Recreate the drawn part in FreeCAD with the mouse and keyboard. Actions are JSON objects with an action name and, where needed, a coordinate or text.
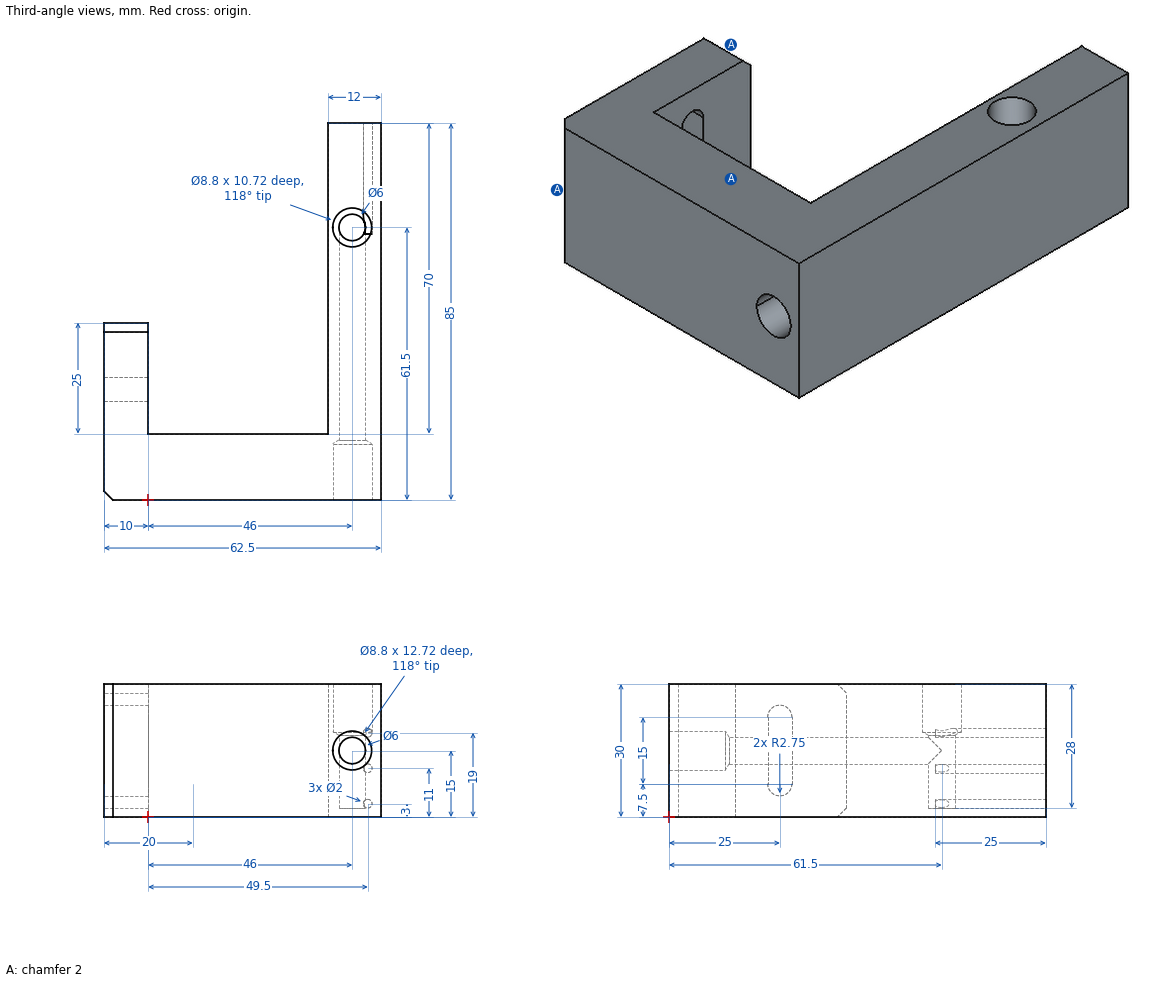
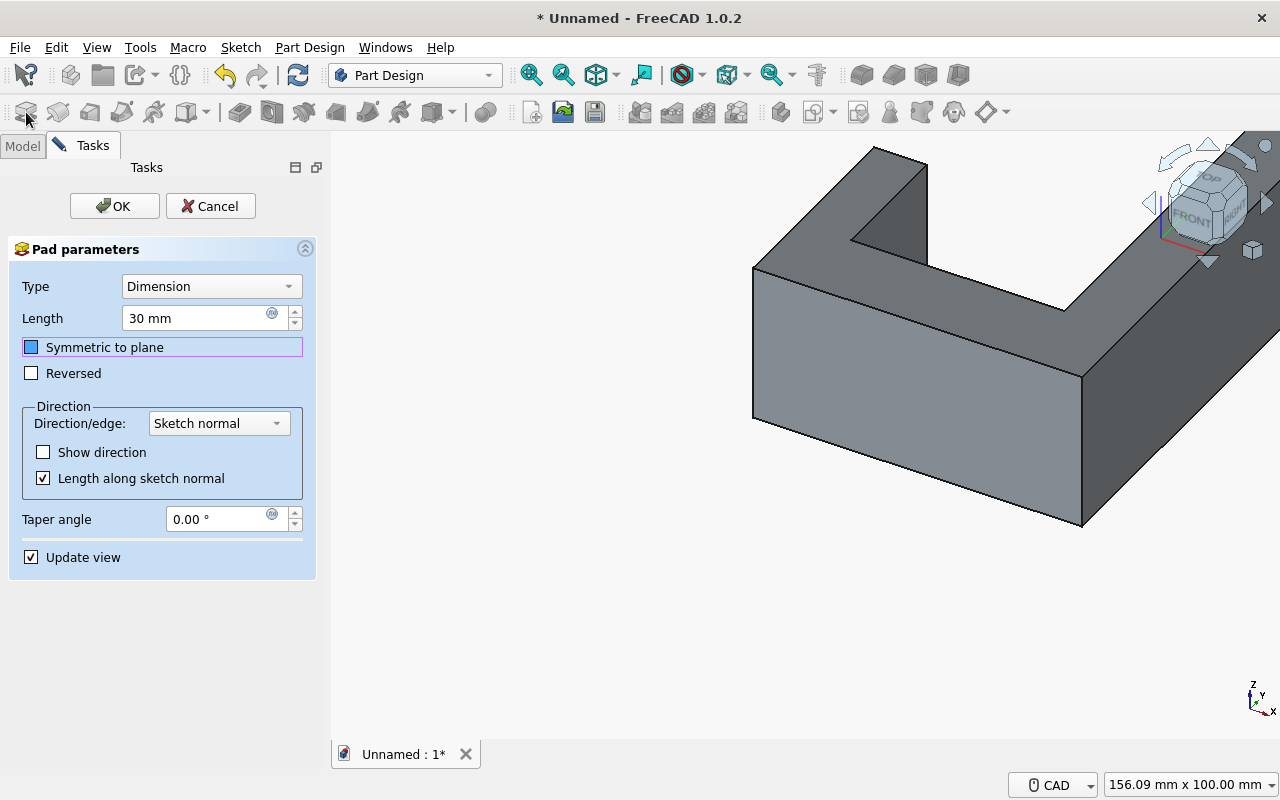
{"action": "left_click", "coordinate": [115, 206]}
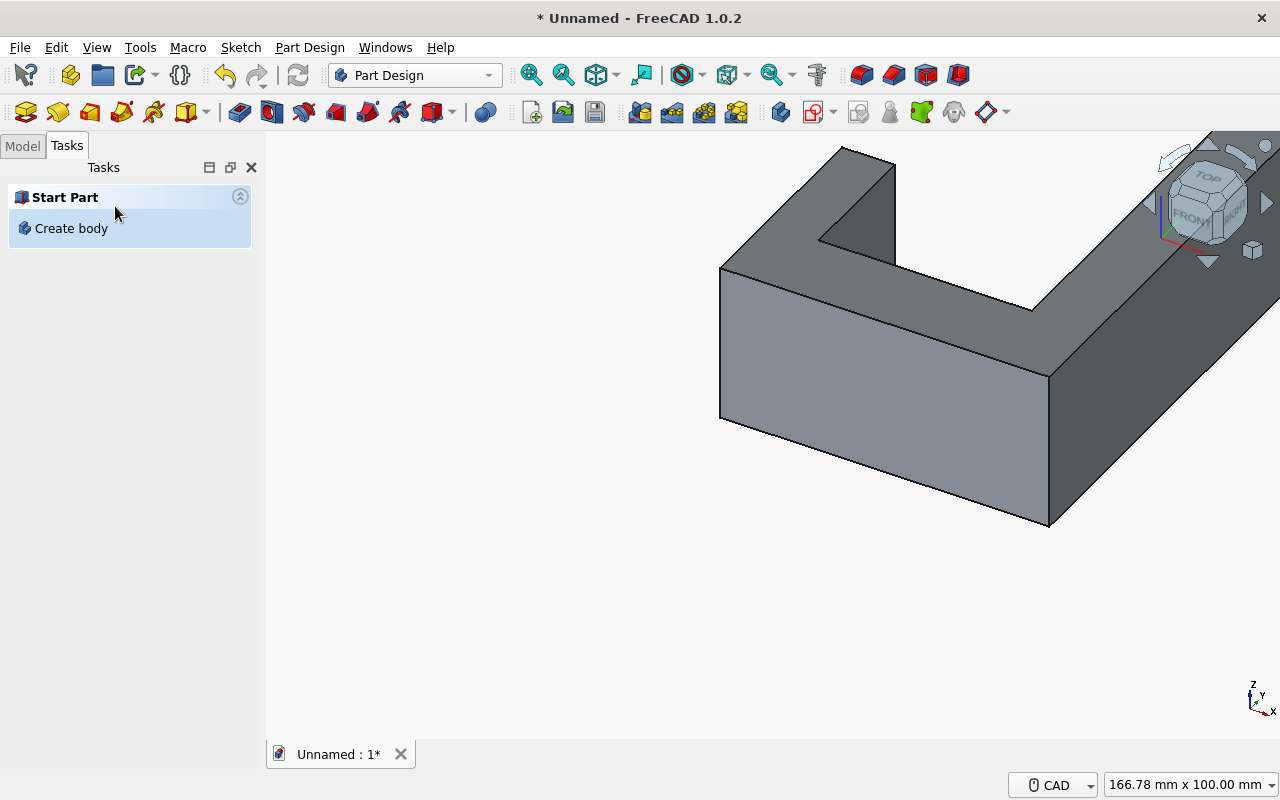
{"action": "key", "text": "v f"}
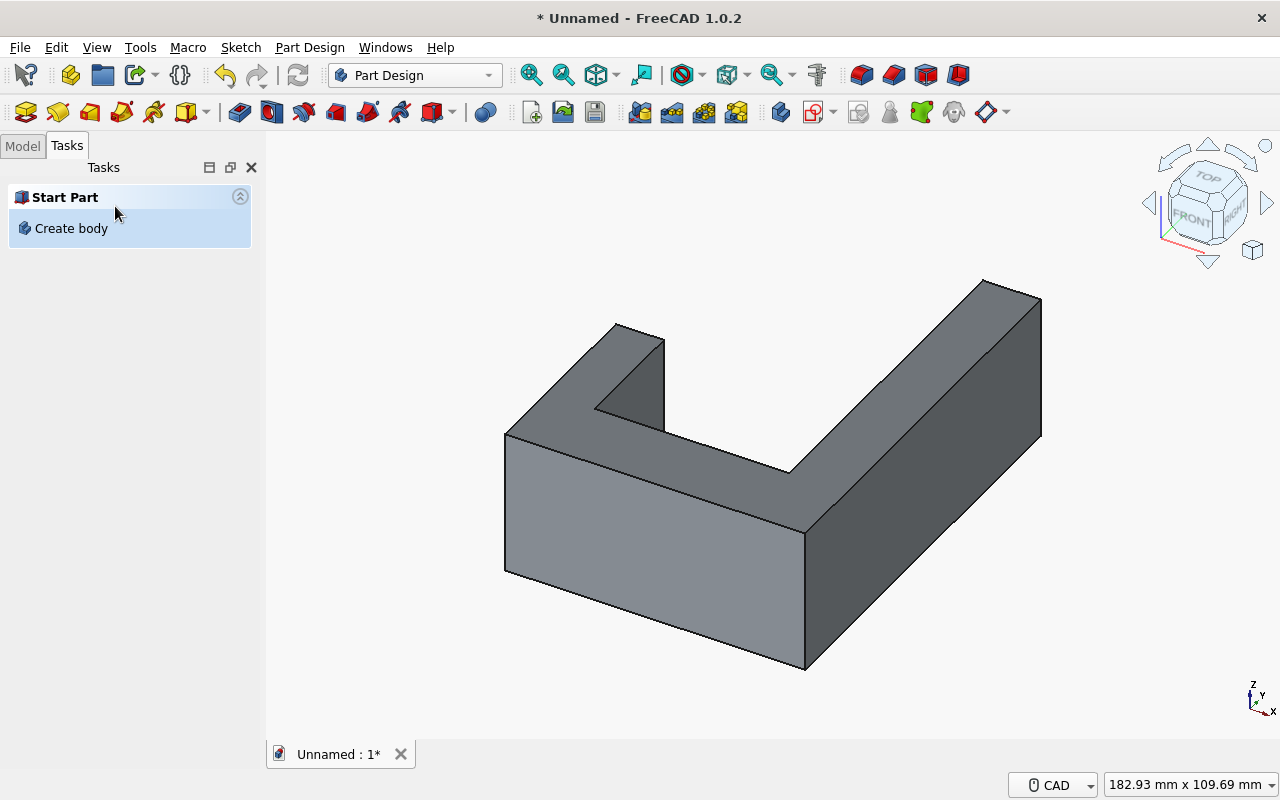
{"action": "key", "text": "4"}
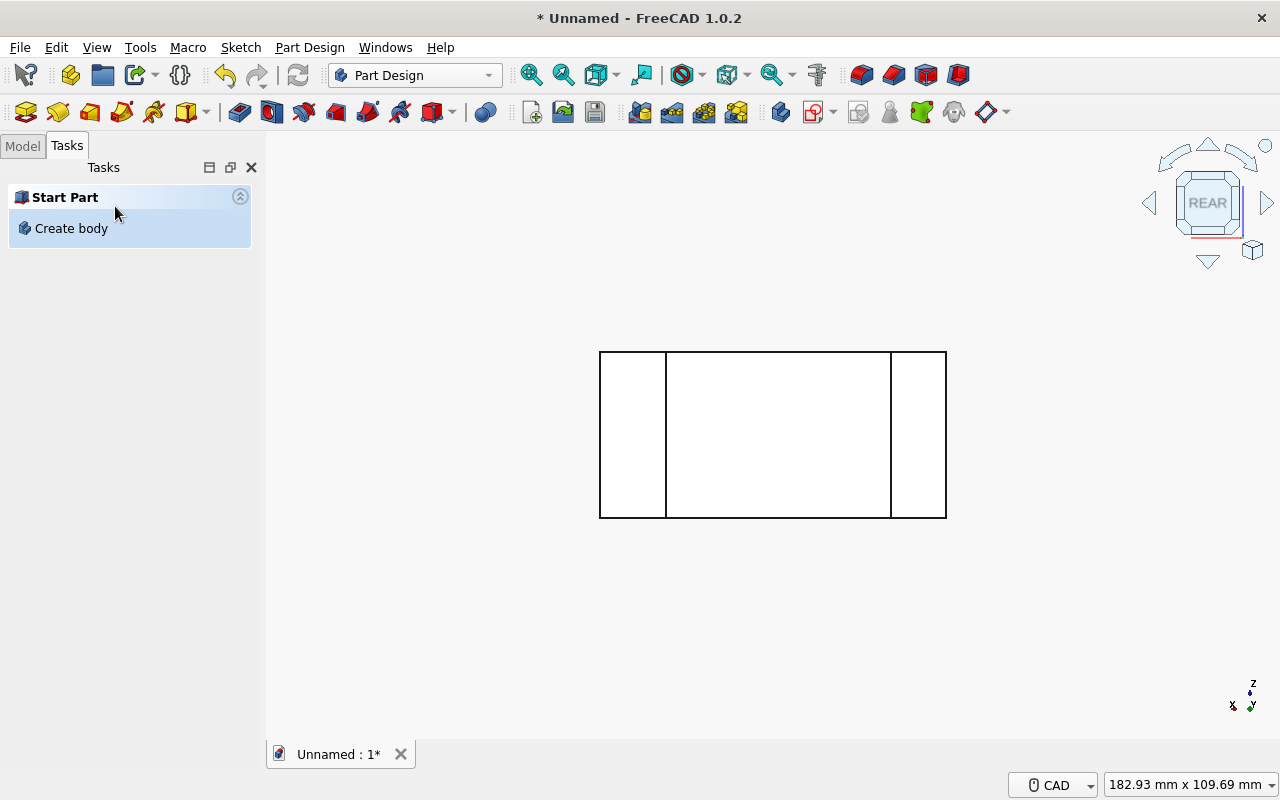
{"action": "key", "text": "v f"}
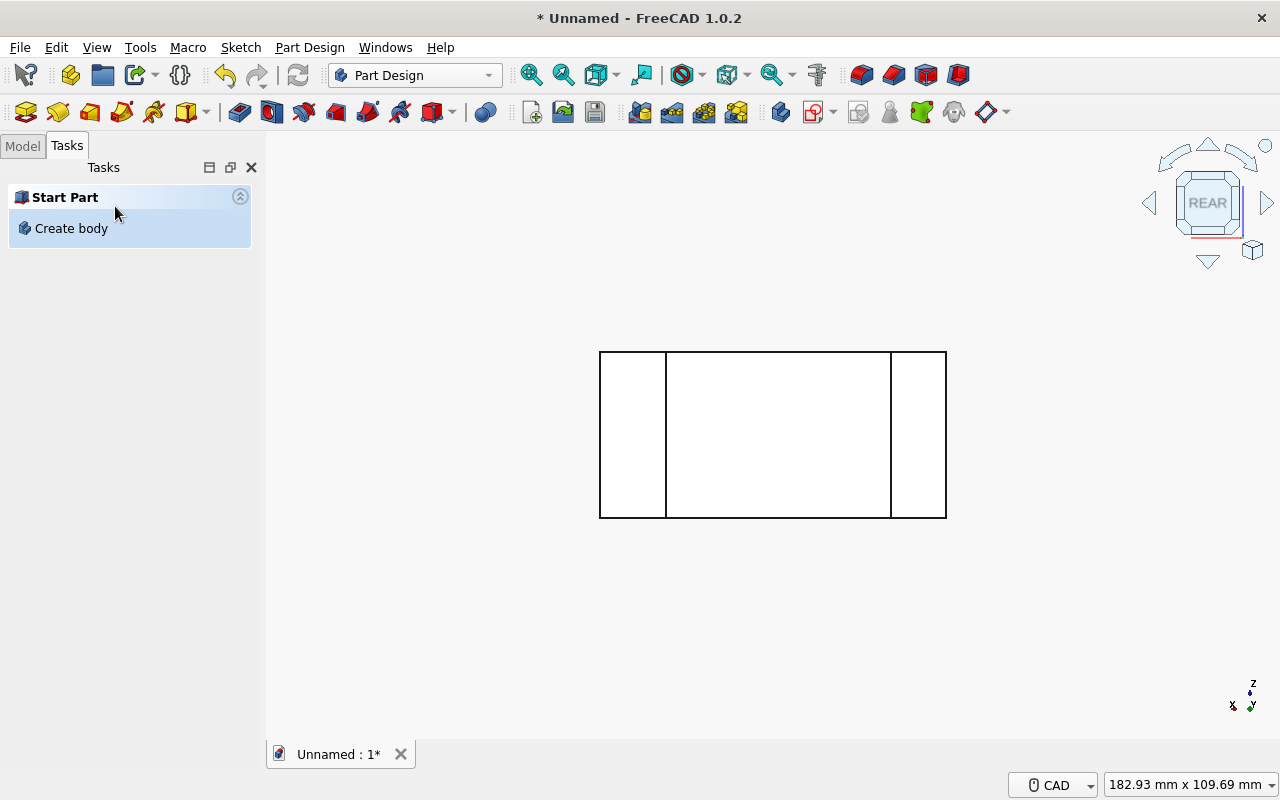
{"action": "left_click", "coordinate": [633, 386]}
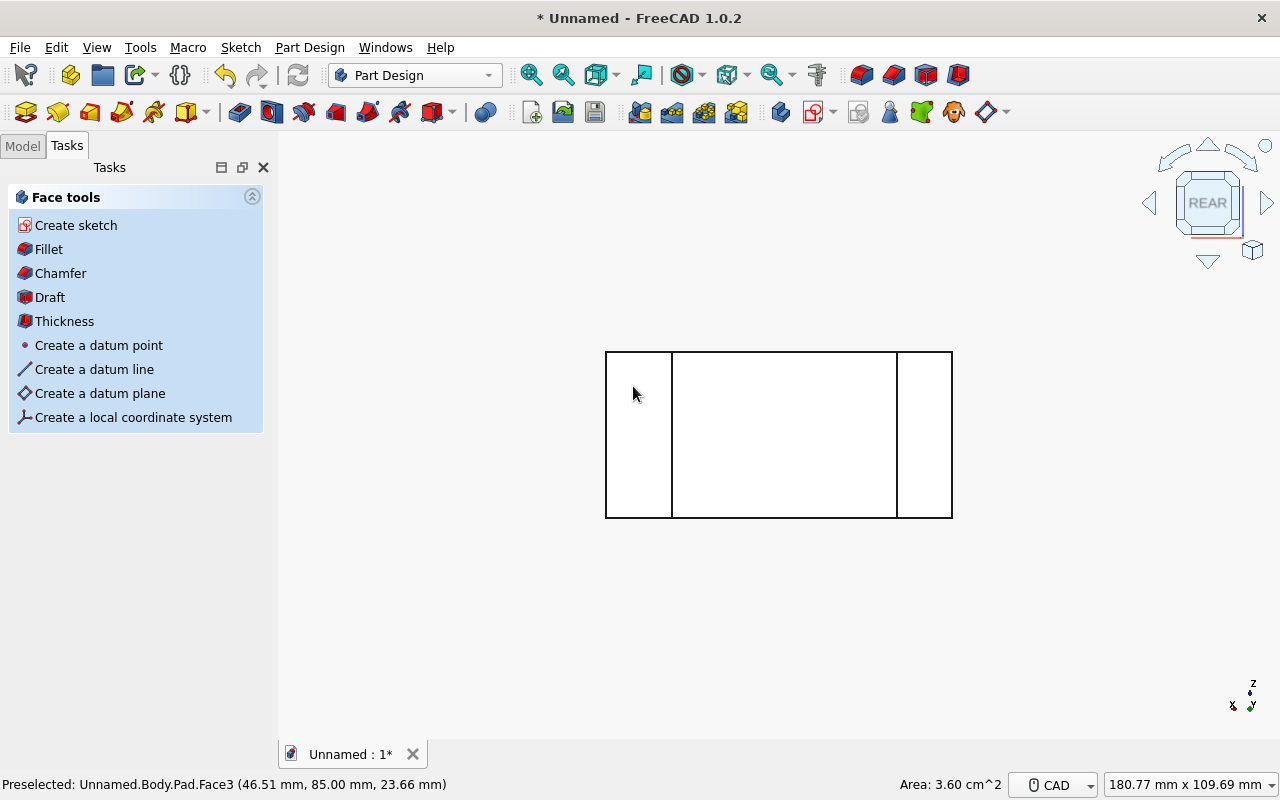
{"action": "left_click", "coordinate": [814, 112]}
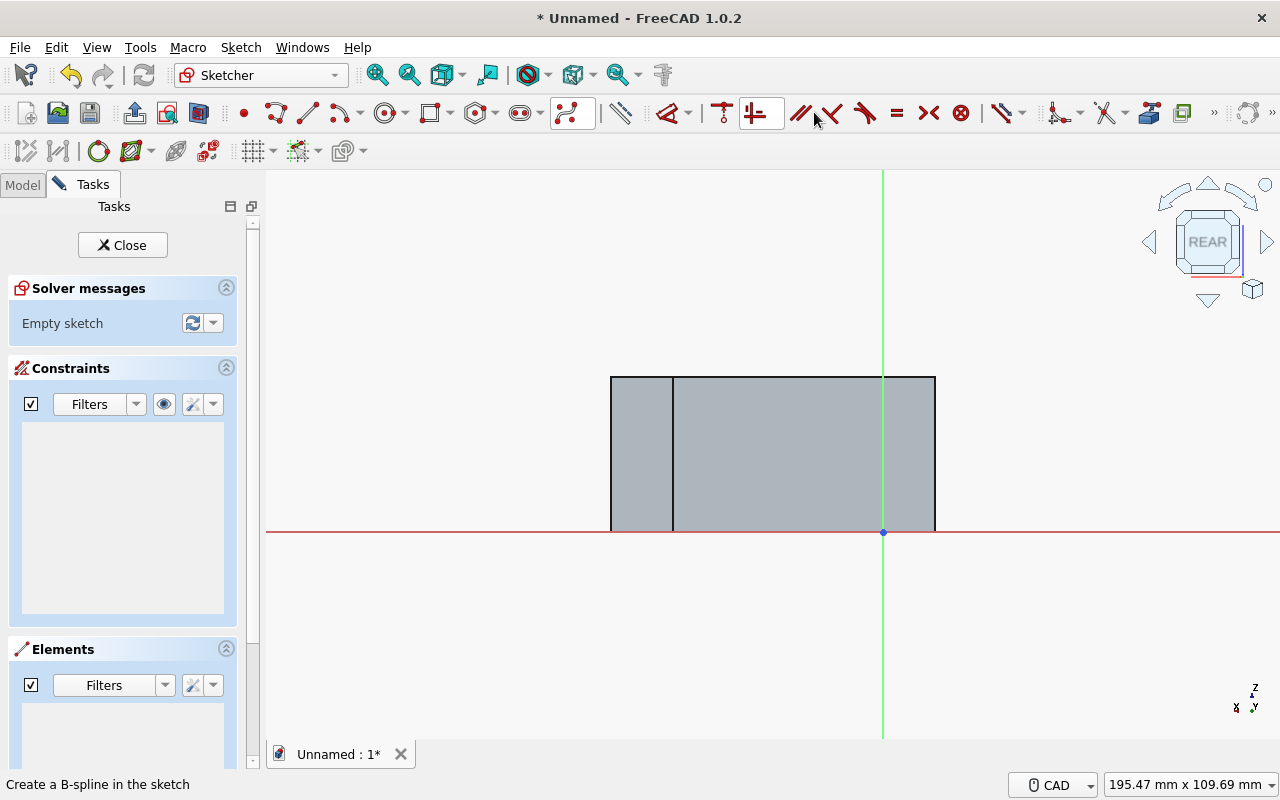
{"action": "scroll", "coordinate": [601, 482], "scroll_direction": "up", "scroll_amount": 7}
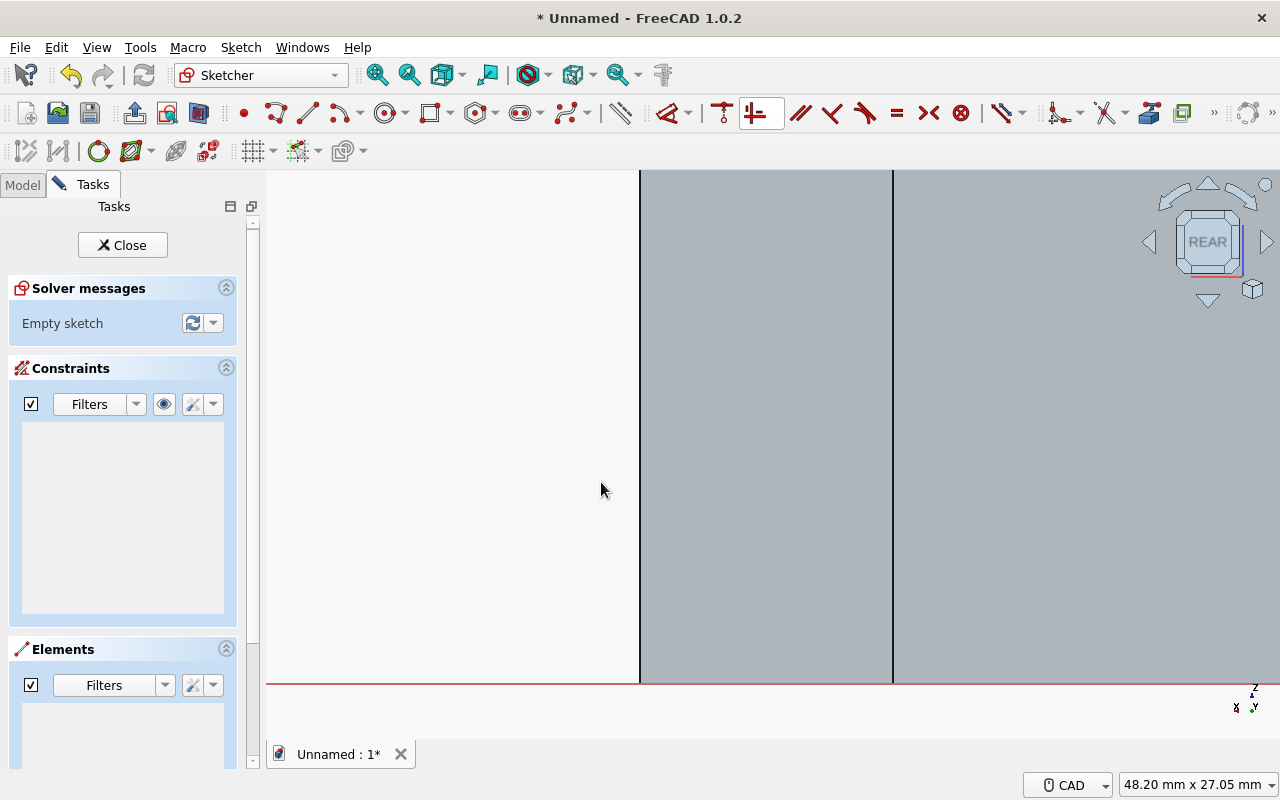
{"action": "left_click", "coordinate": [386, 114]}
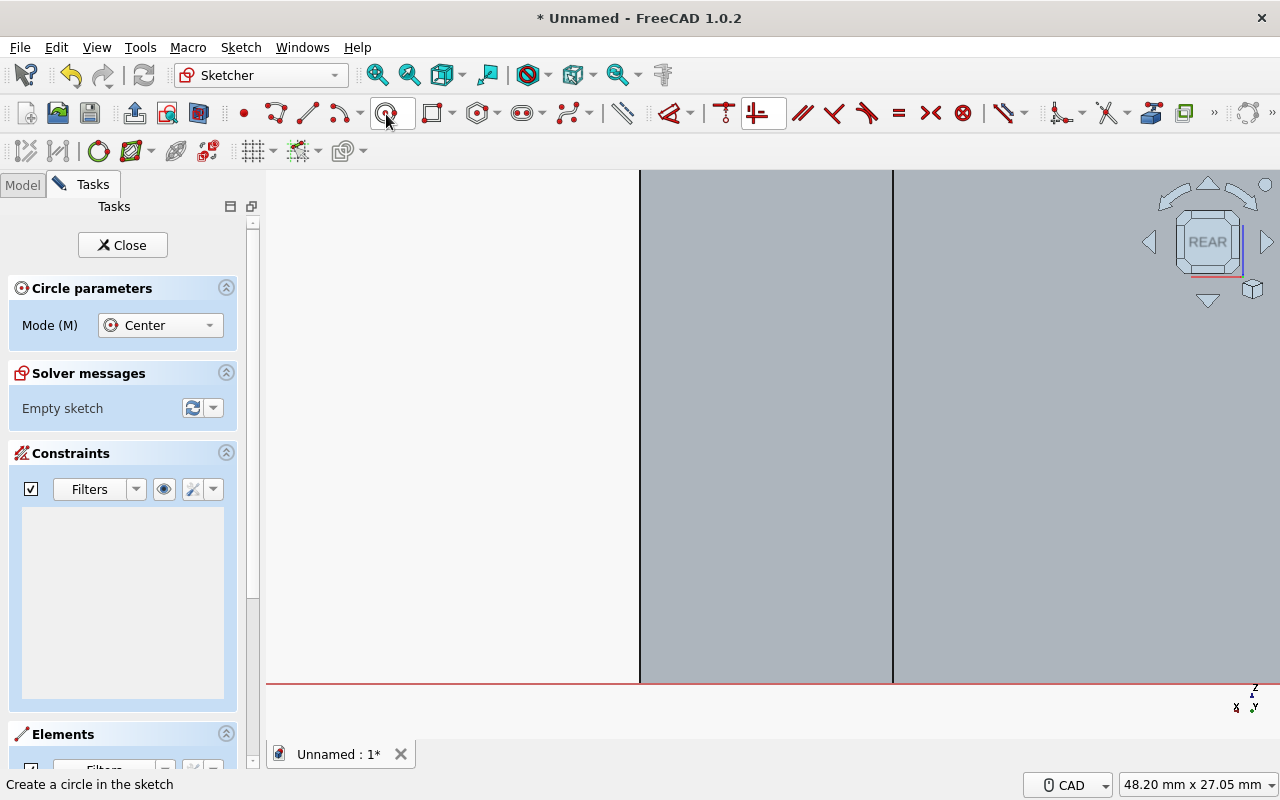
{"action": "left_click", "coordinate": [703, 621]}
{"action": "mouse_move", "coordinate": [718, 606]}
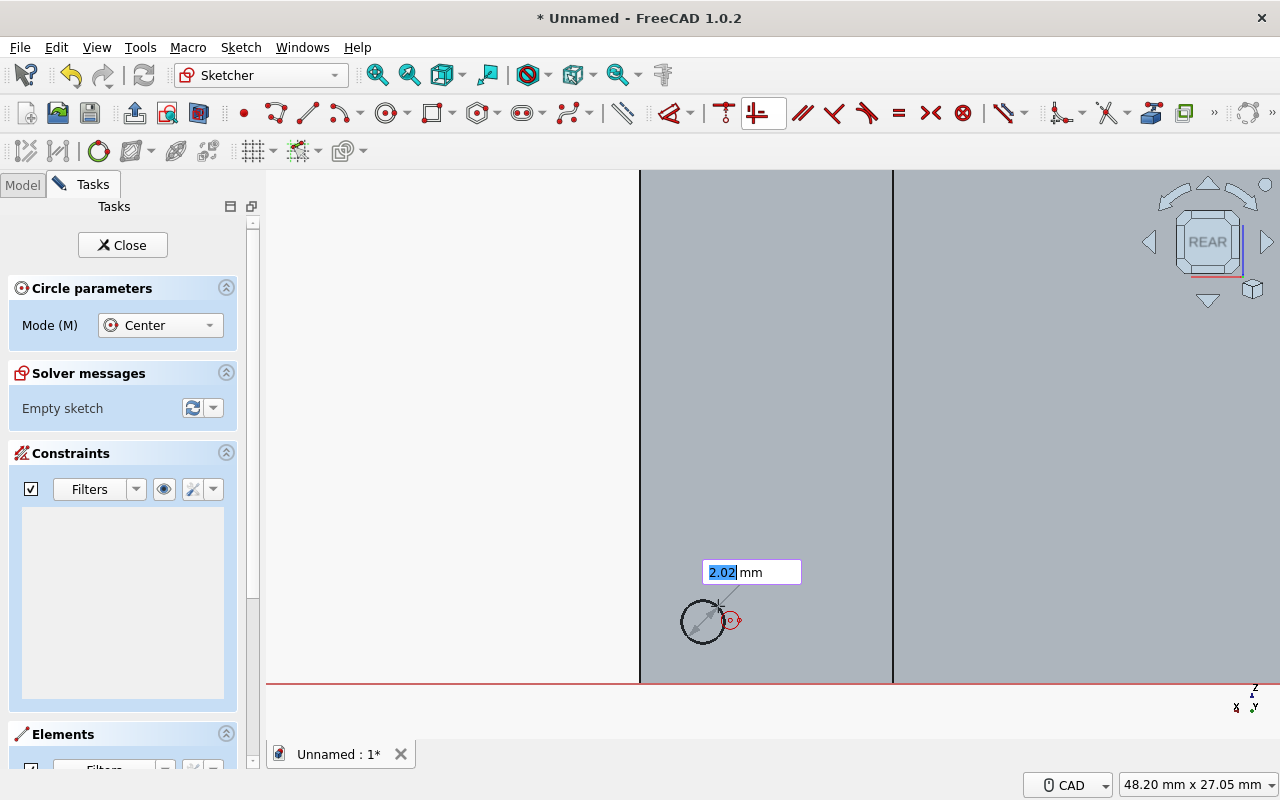
{"action": "type", "text": "2"}
{"action": "key", "text": "Return"}